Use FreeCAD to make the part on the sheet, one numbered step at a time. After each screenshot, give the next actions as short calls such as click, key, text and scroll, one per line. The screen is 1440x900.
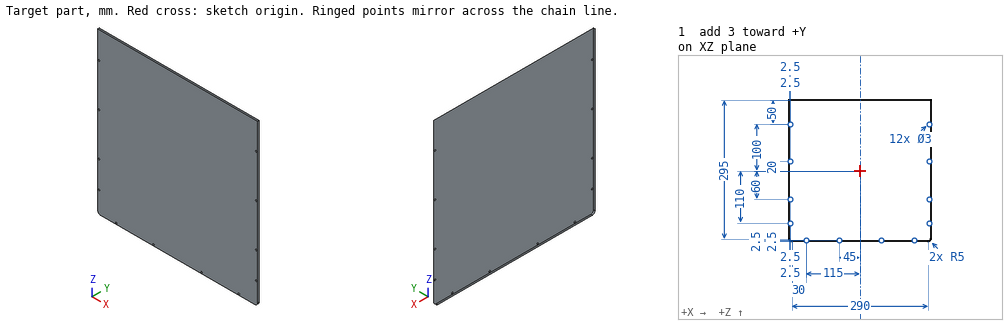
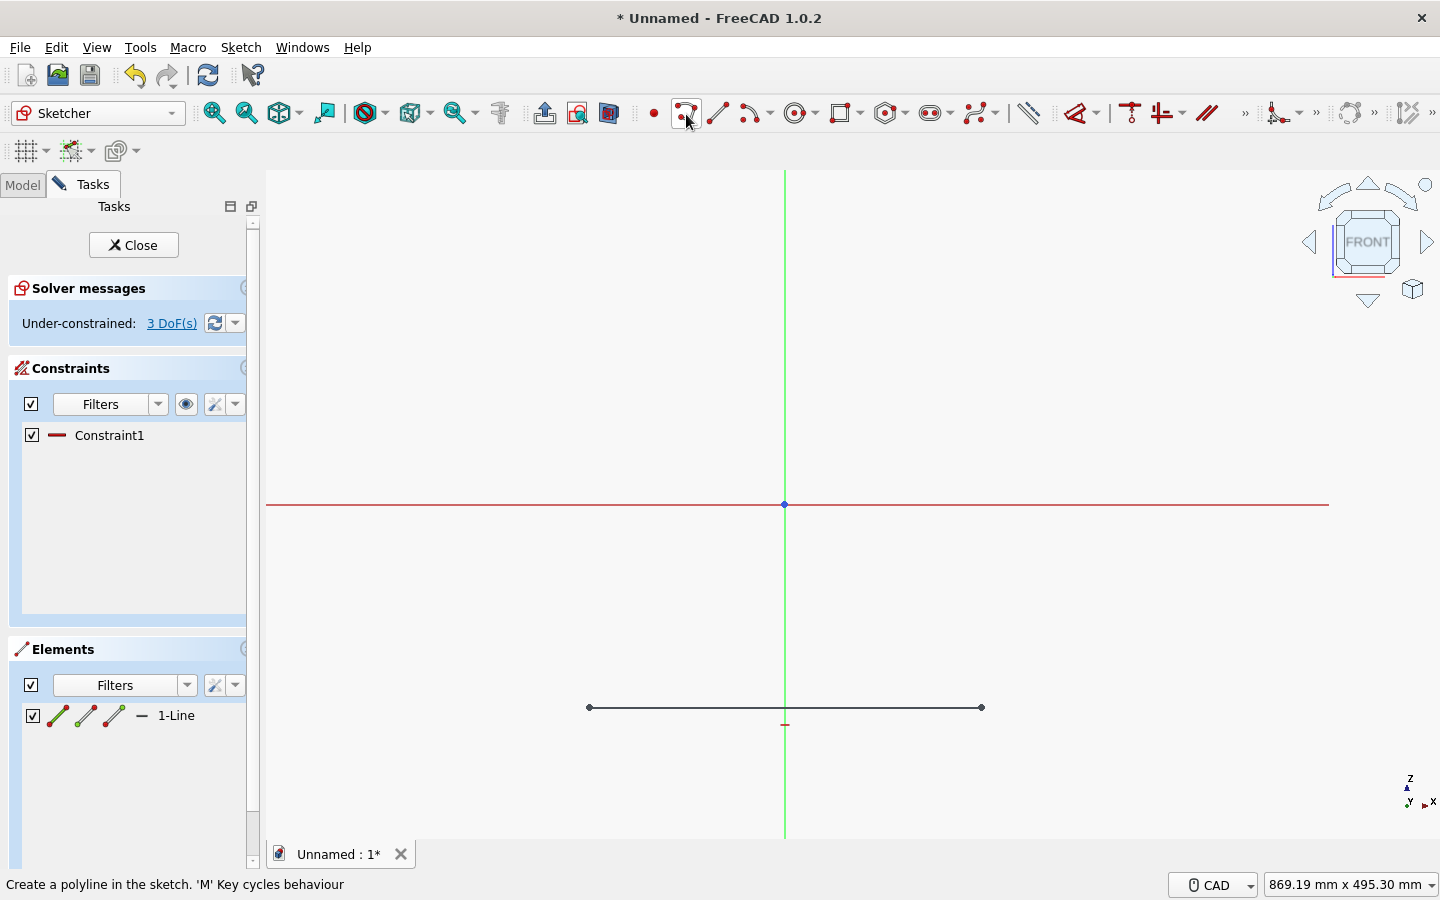
scroll(582, 700, up, 3)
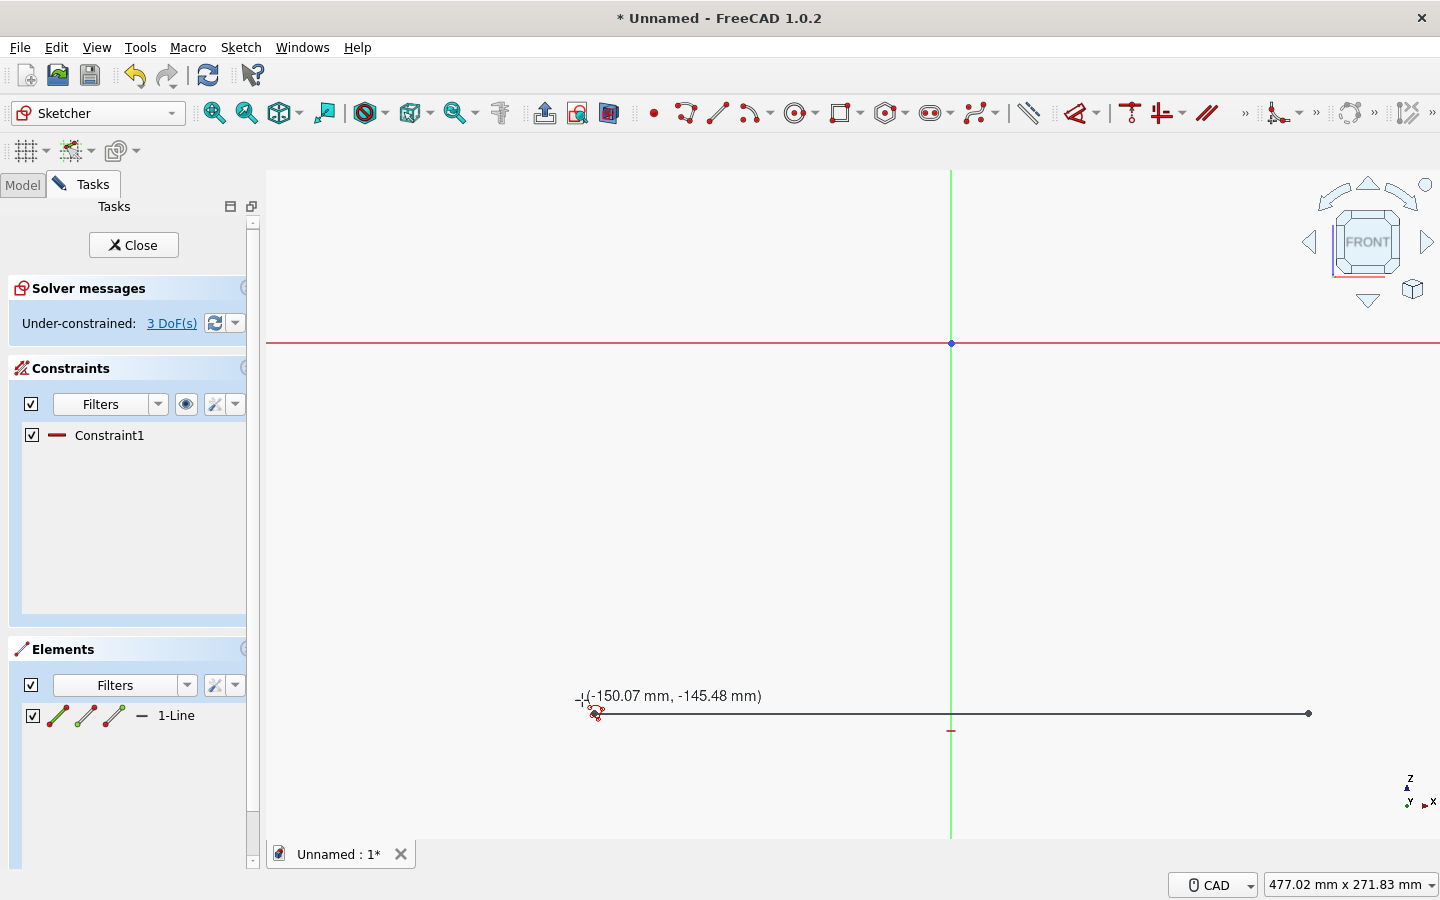
click(582, 700)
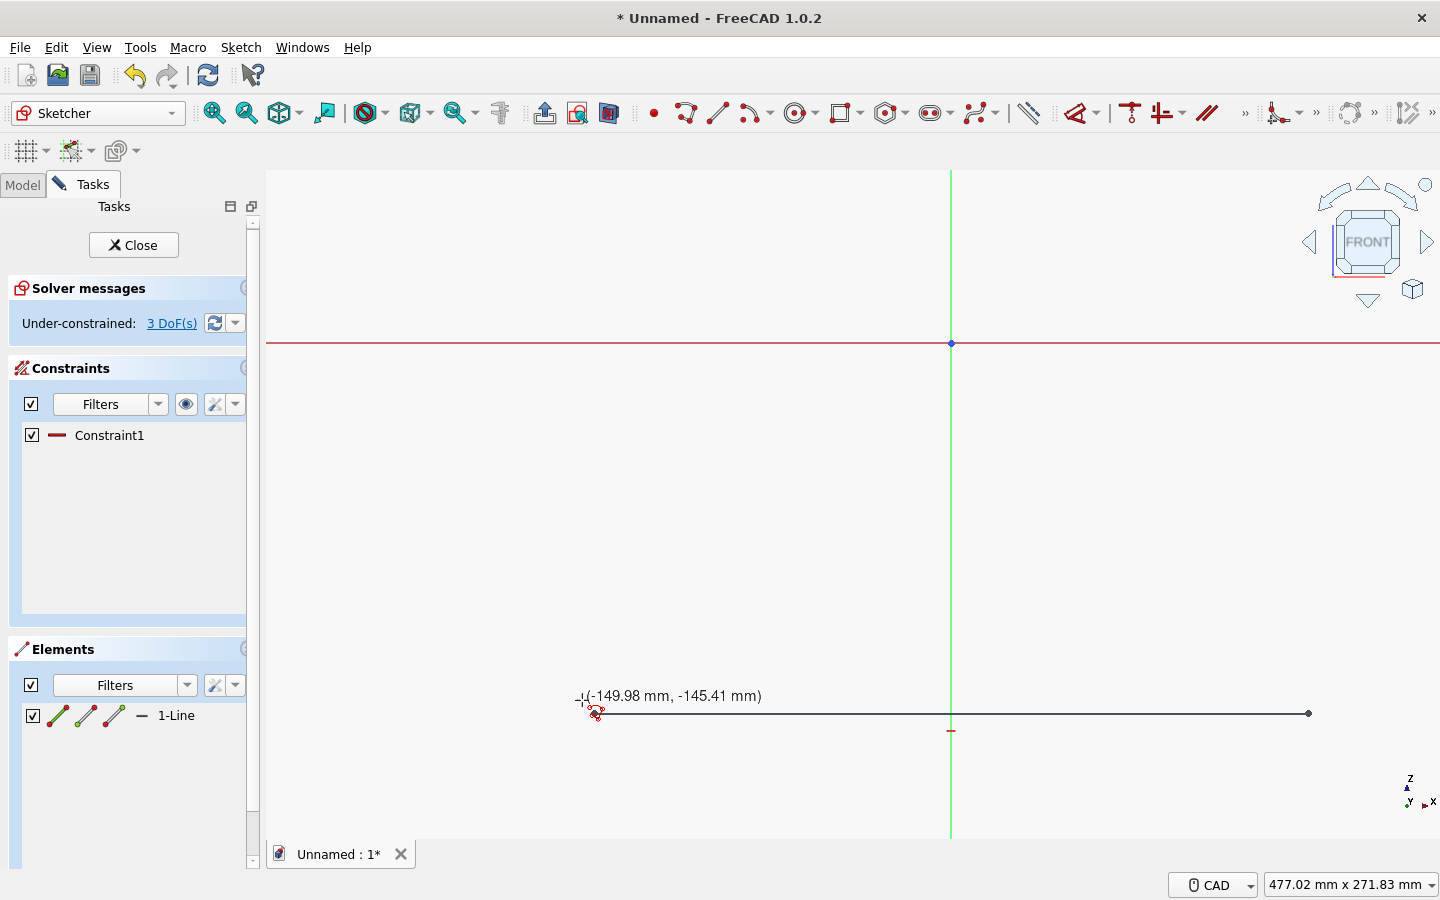
scroll(582, 701, down, 3)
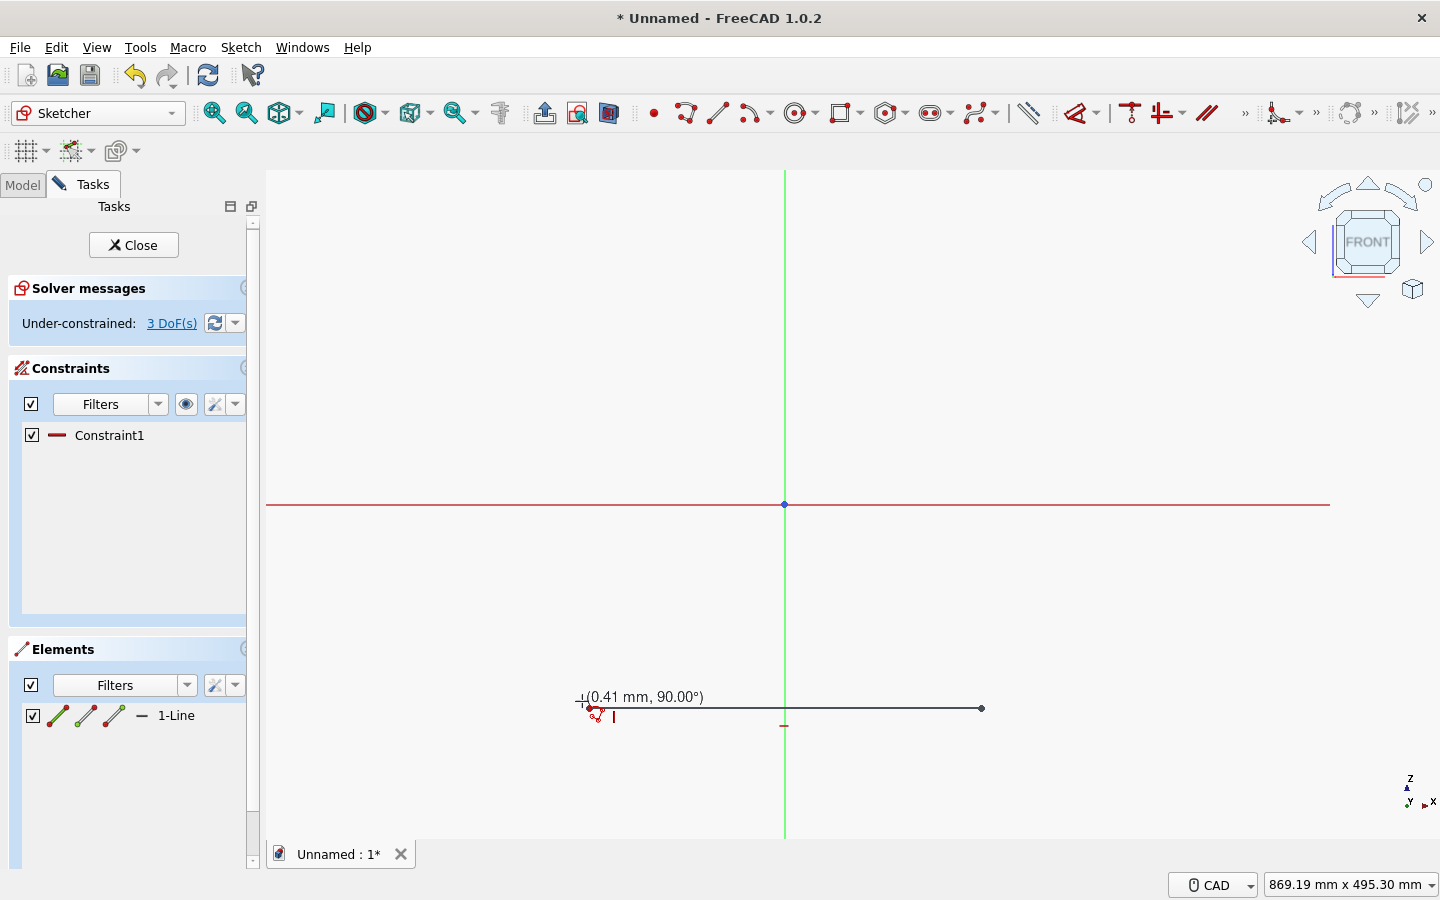
click(582, 302)
click(987, 302)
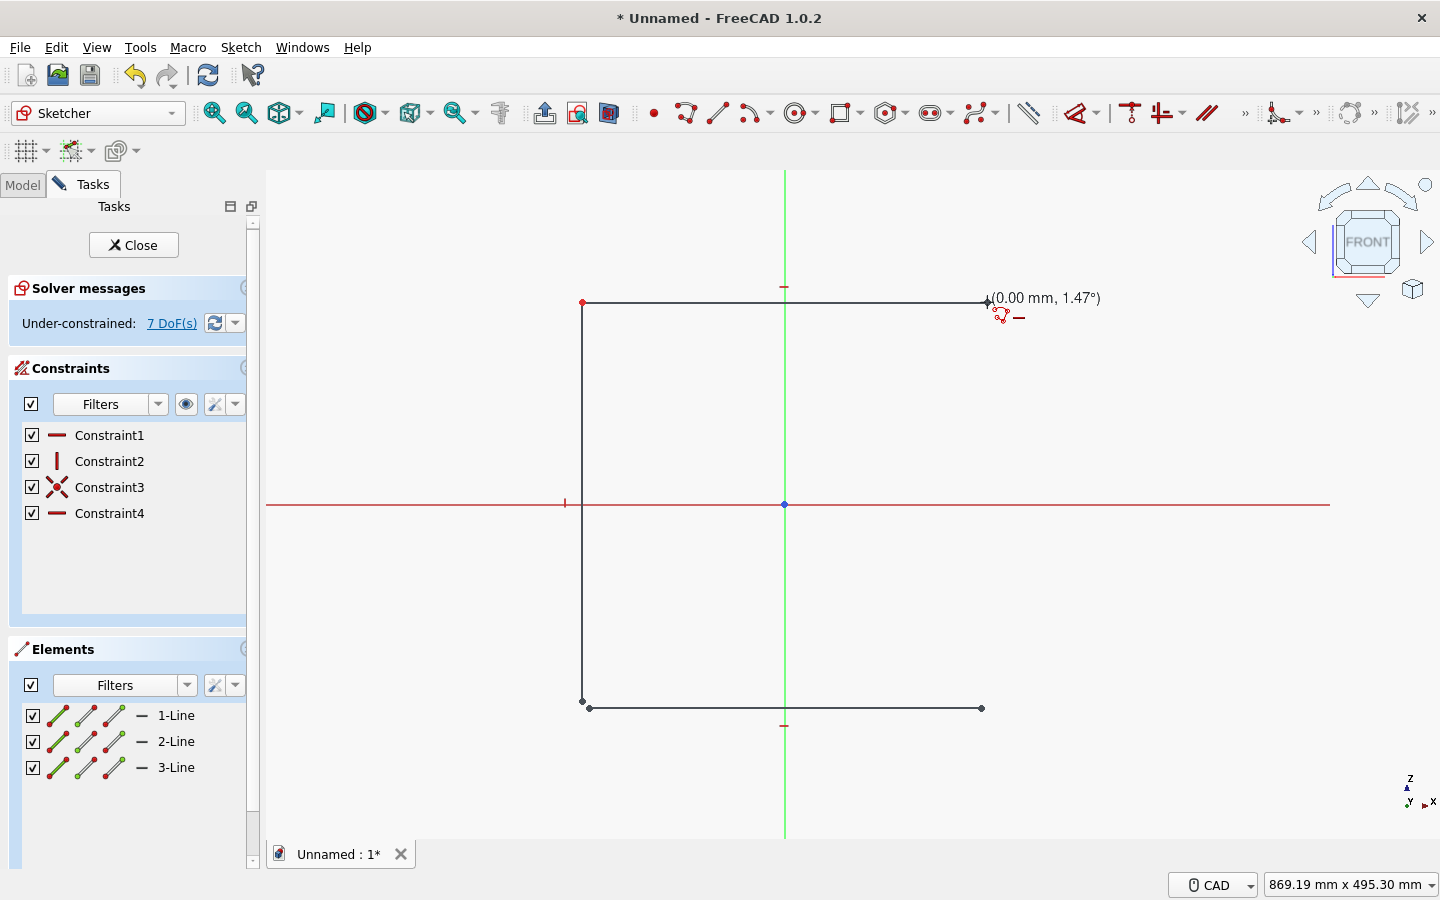
scroll(987, 701, up, 3)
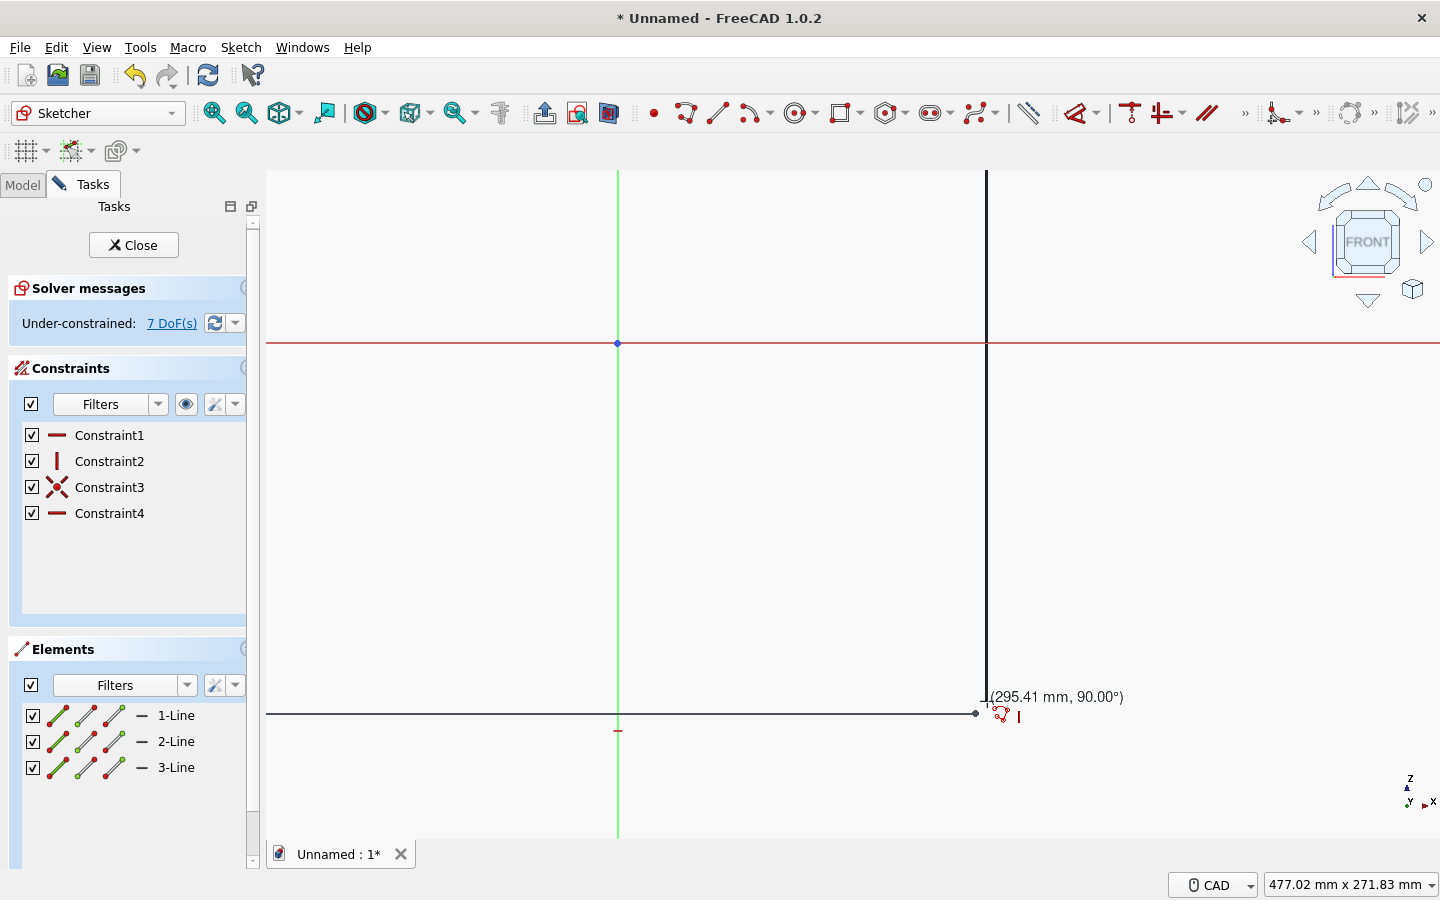
click(986, 700)
right_click(986, 700)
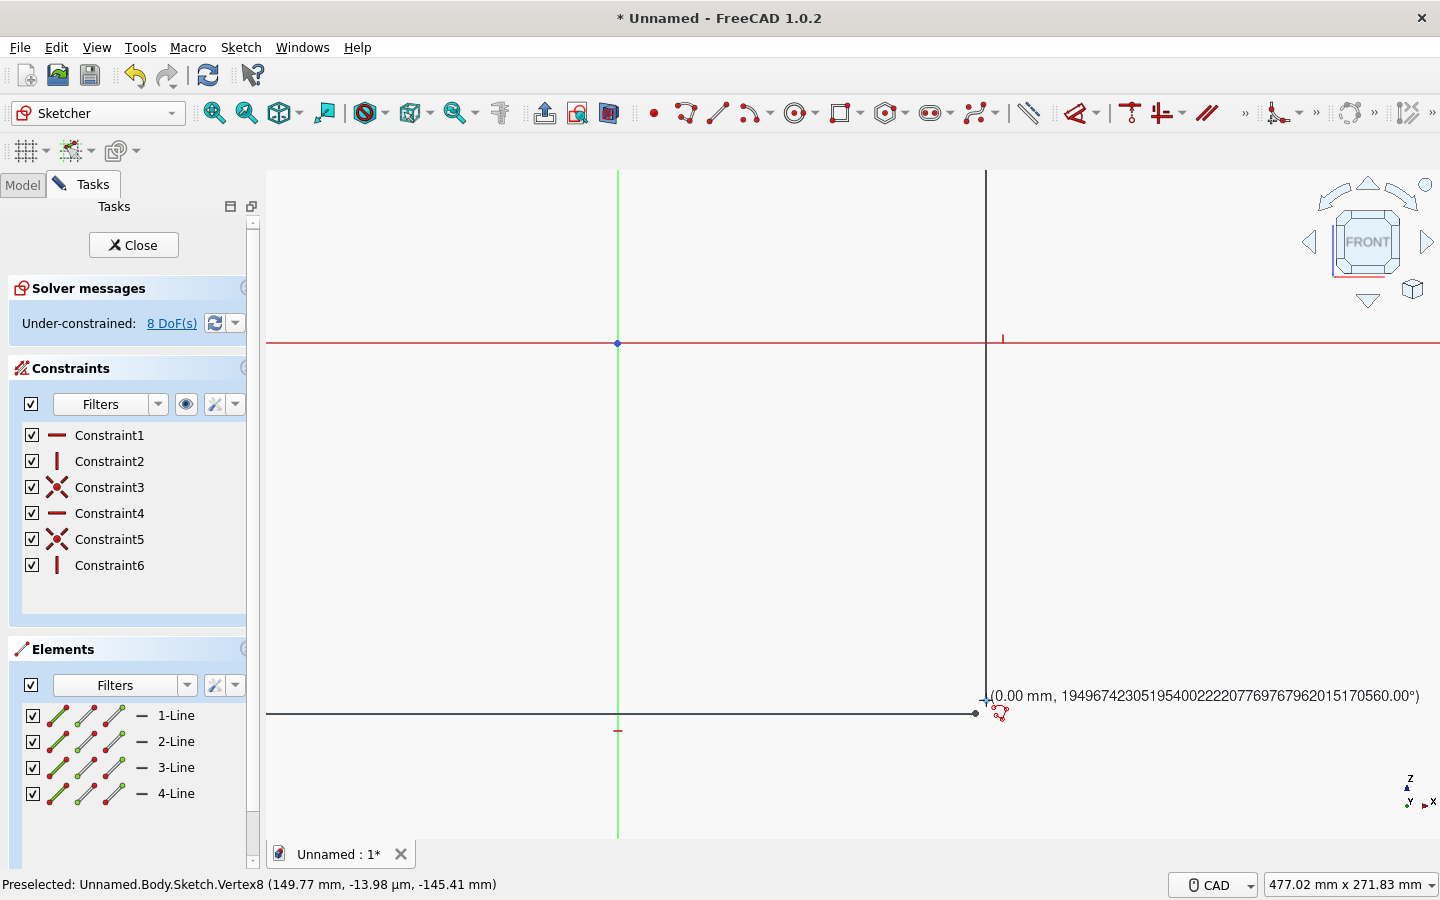
click(772, 114)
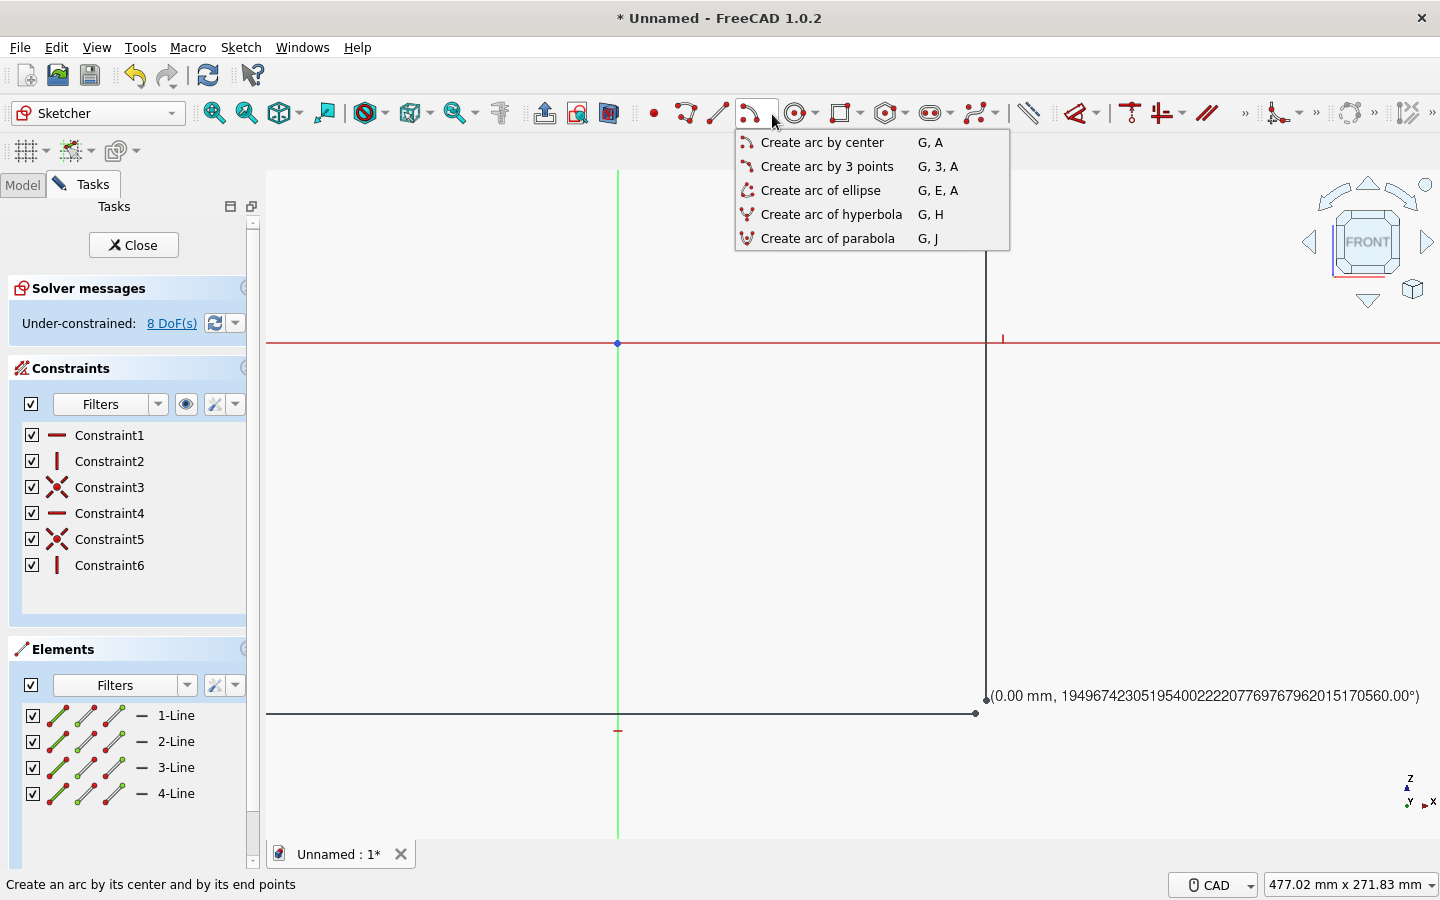
click(872, 166)